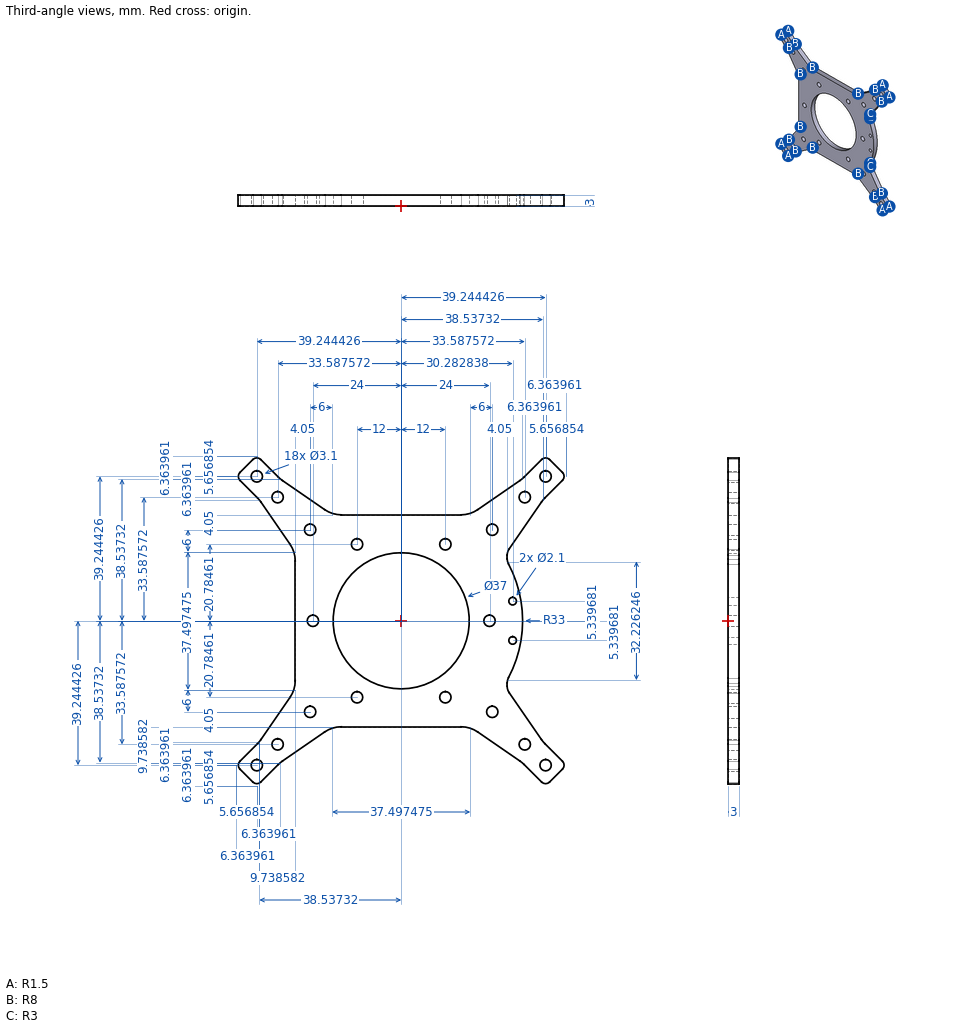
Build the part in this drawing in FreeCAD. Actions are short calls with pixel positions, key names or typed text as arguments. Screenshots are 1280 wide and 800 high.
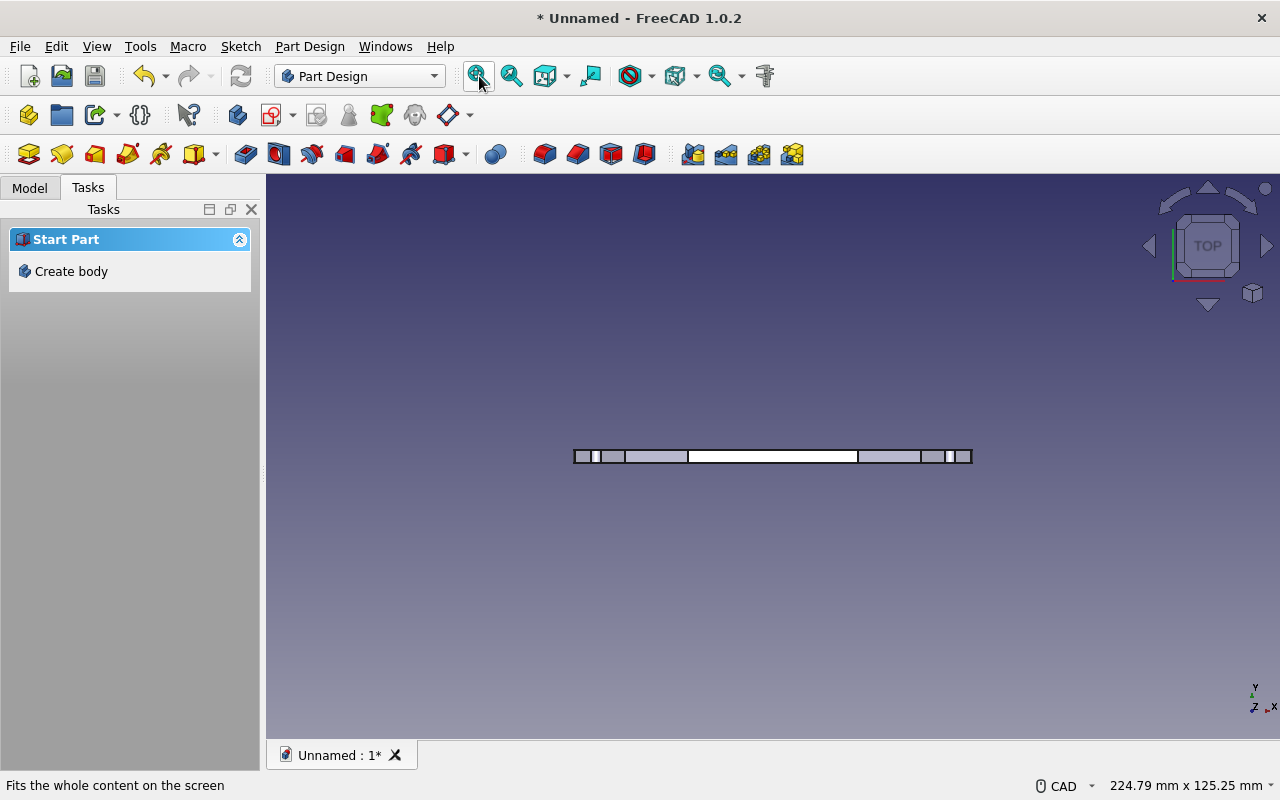
click(479, 76)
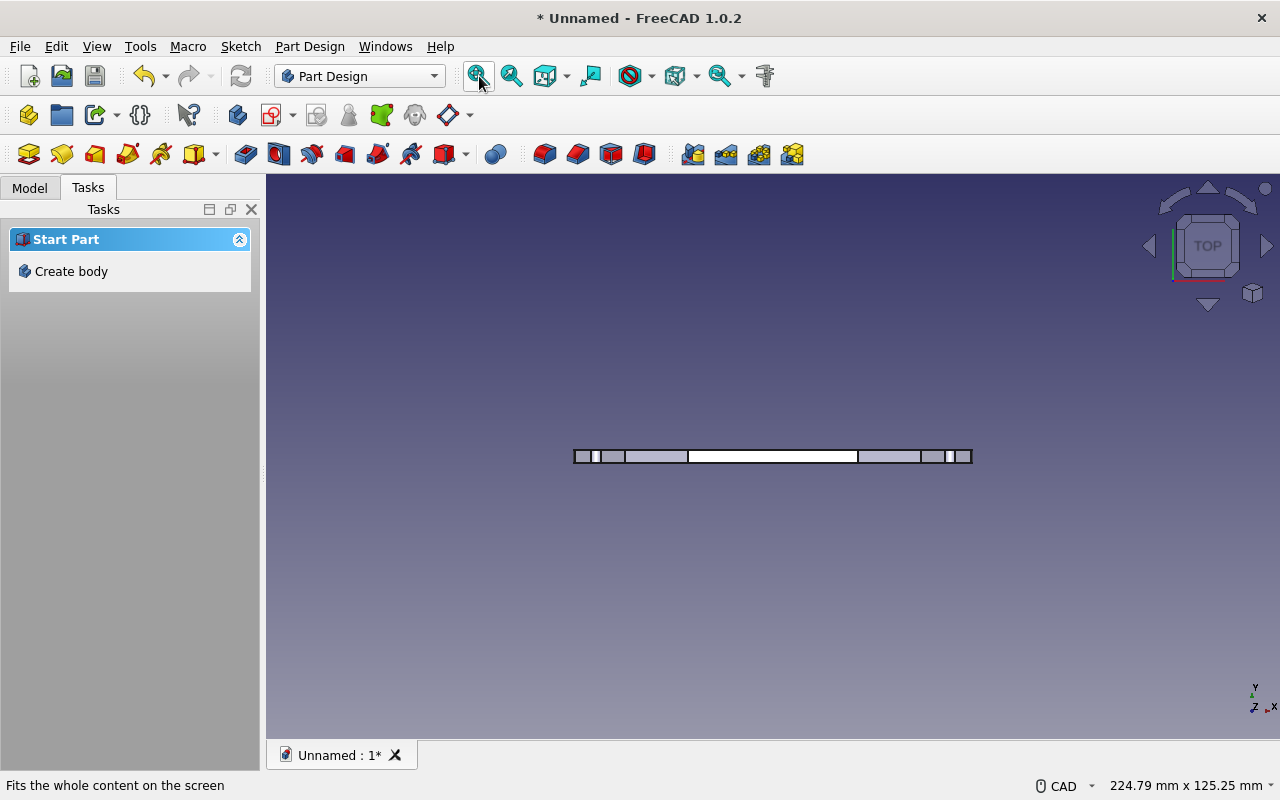
scroll(858, 455, up, 6)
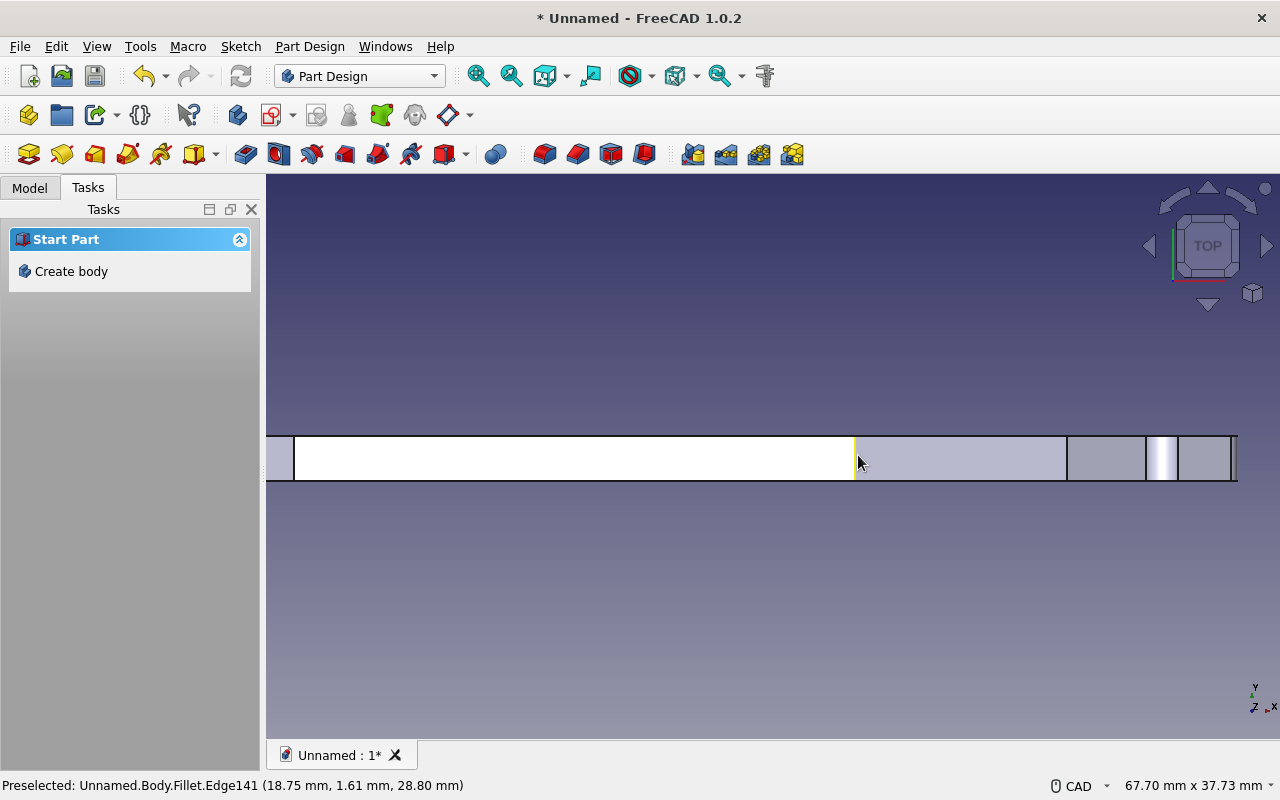
click(479, 76)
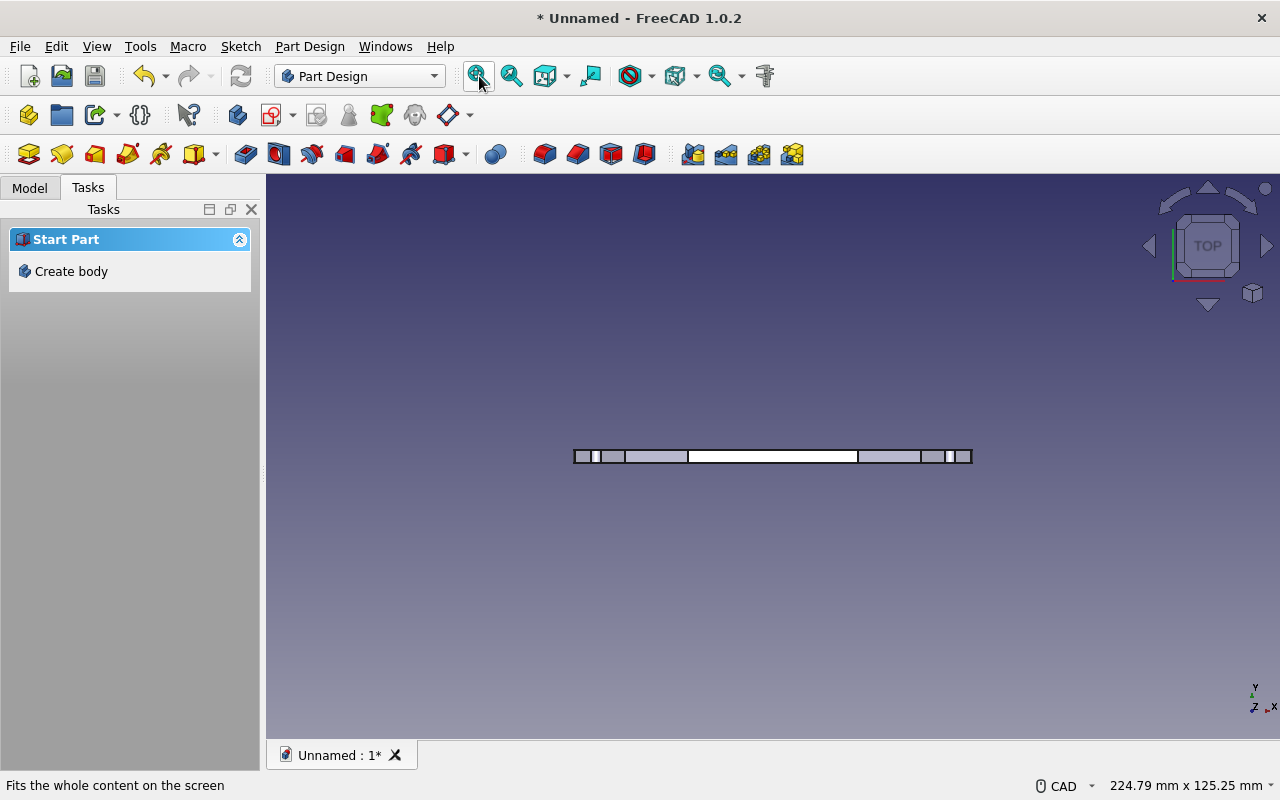
key(1)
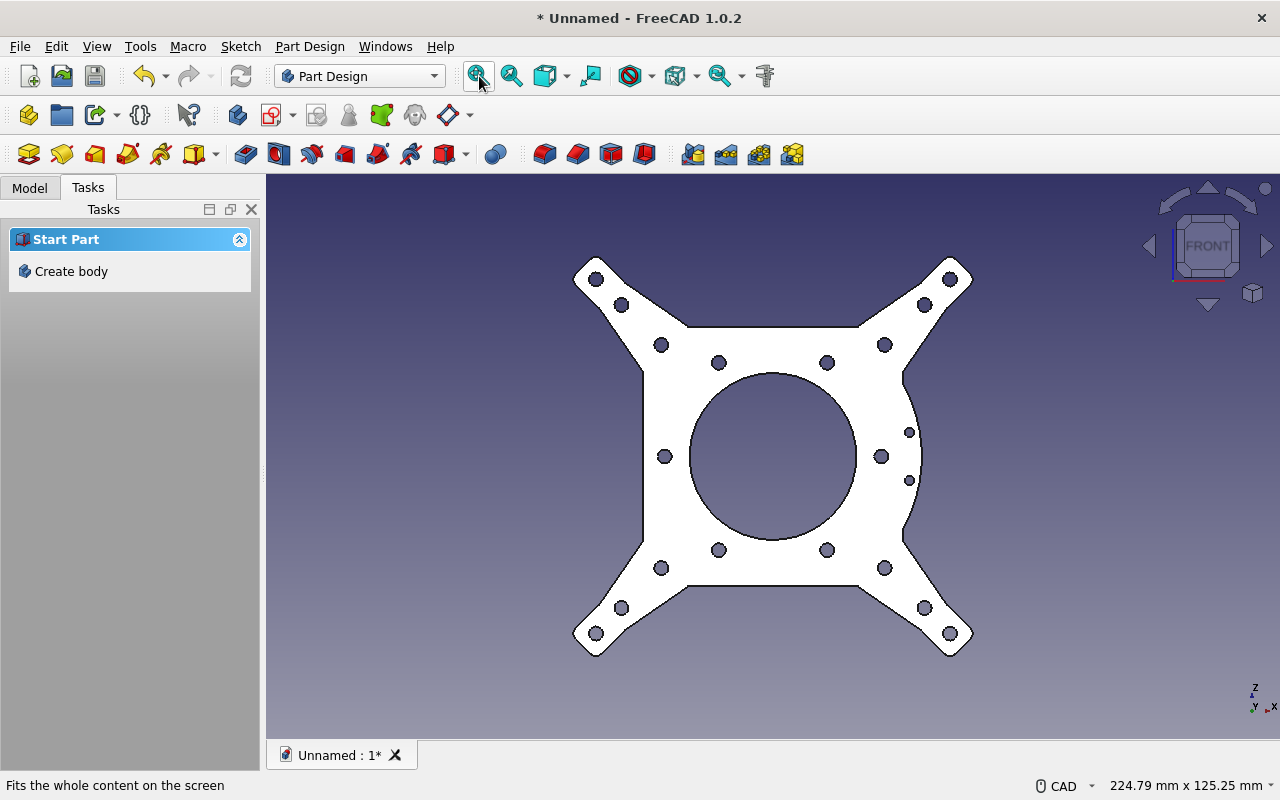
scroll(858, 585, up, 6)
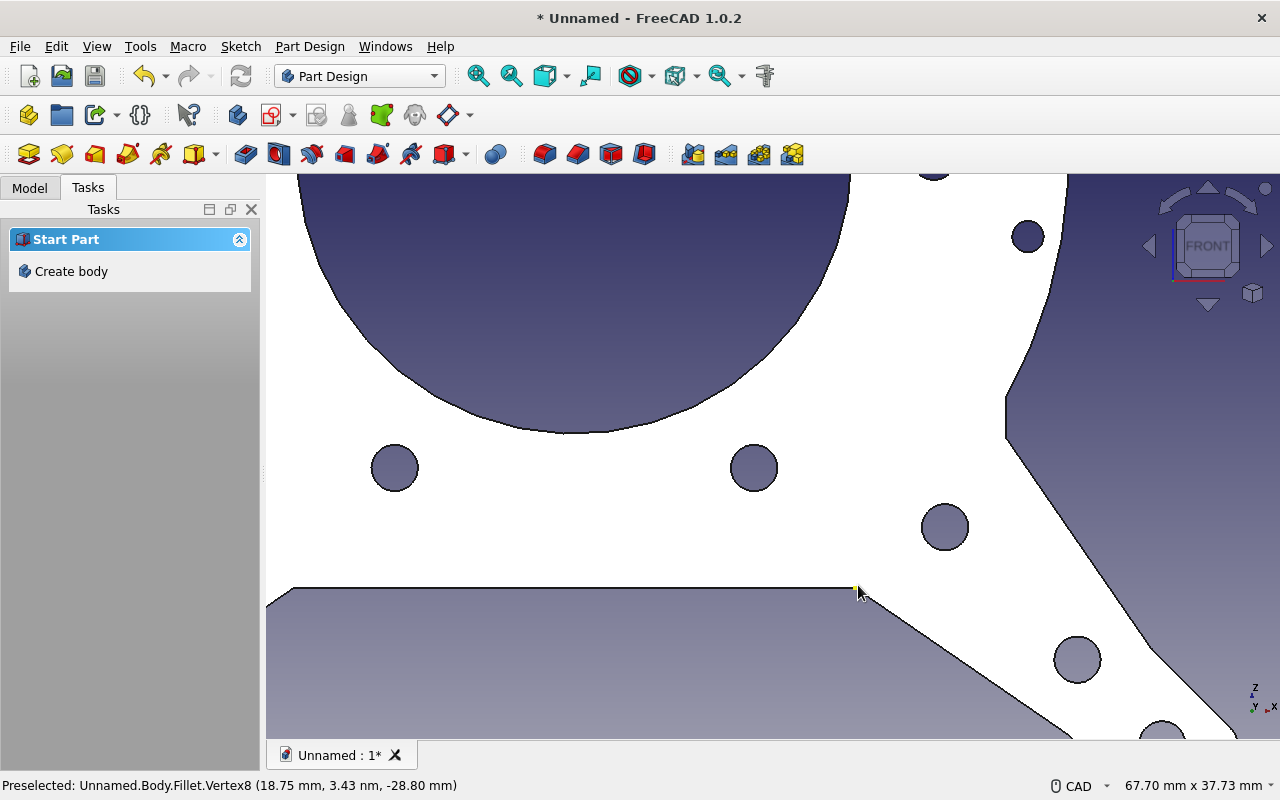
click(479, 76)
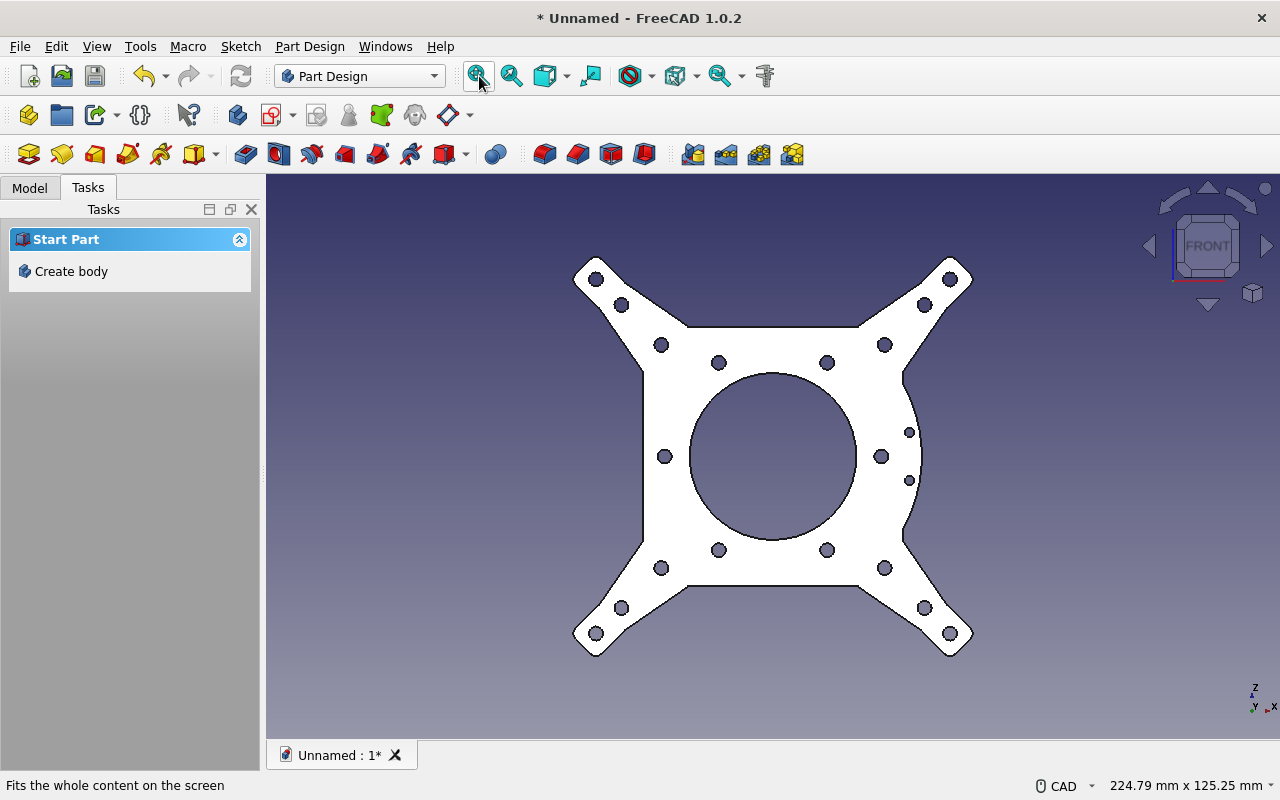
key(3)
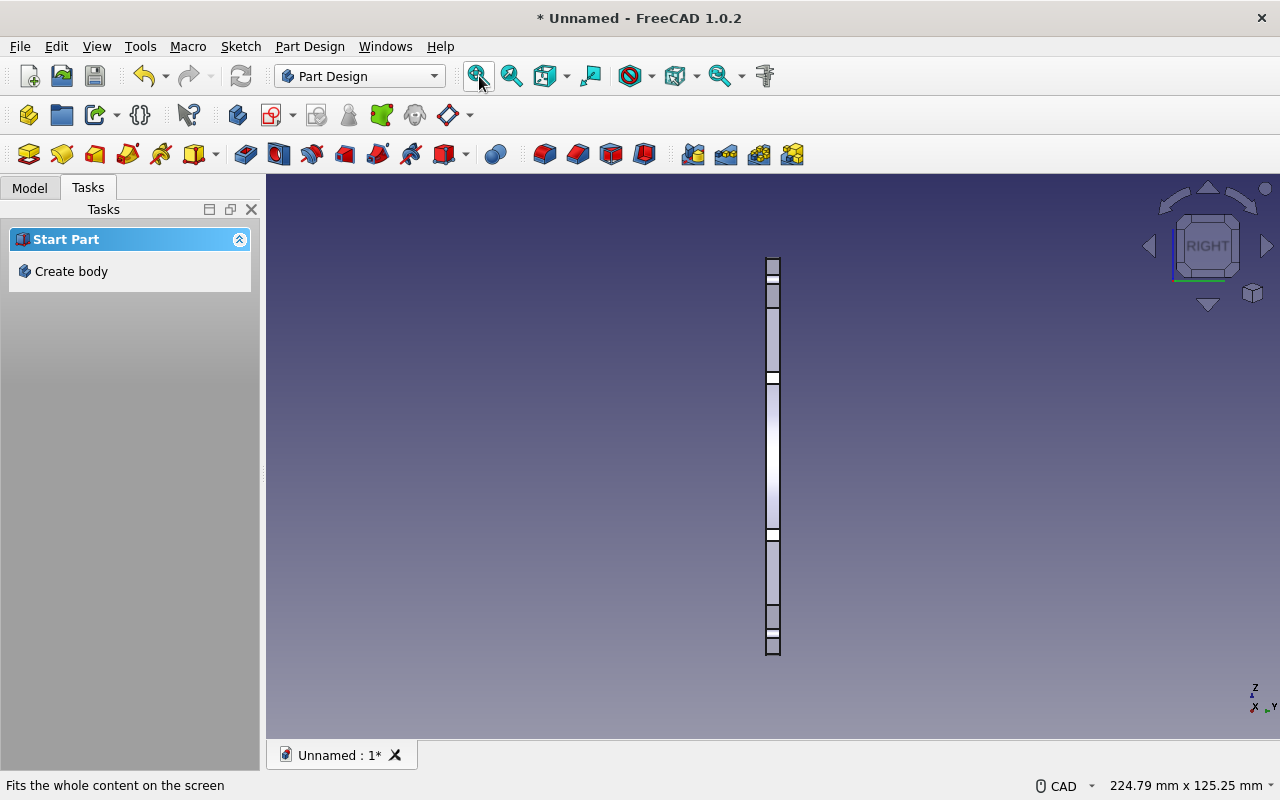
scroll(773, 585, up, 6)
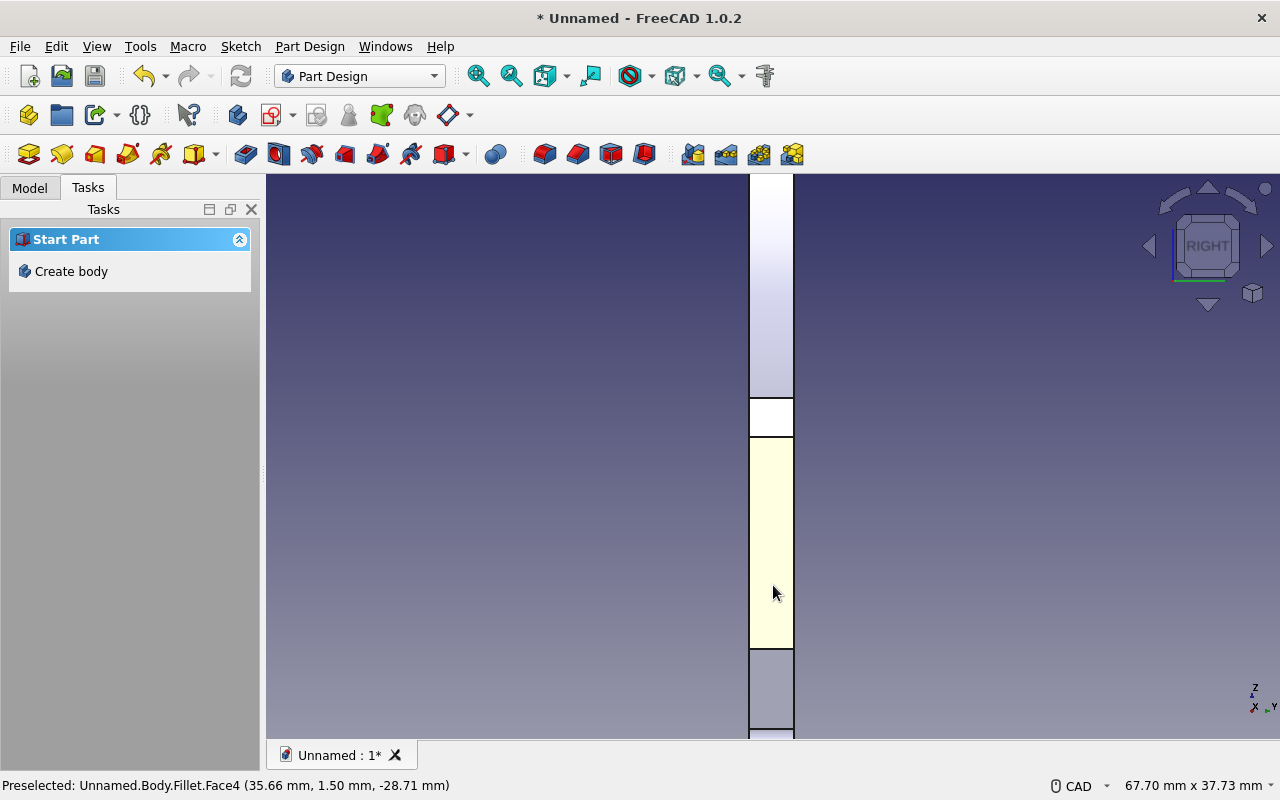
click(479, 76)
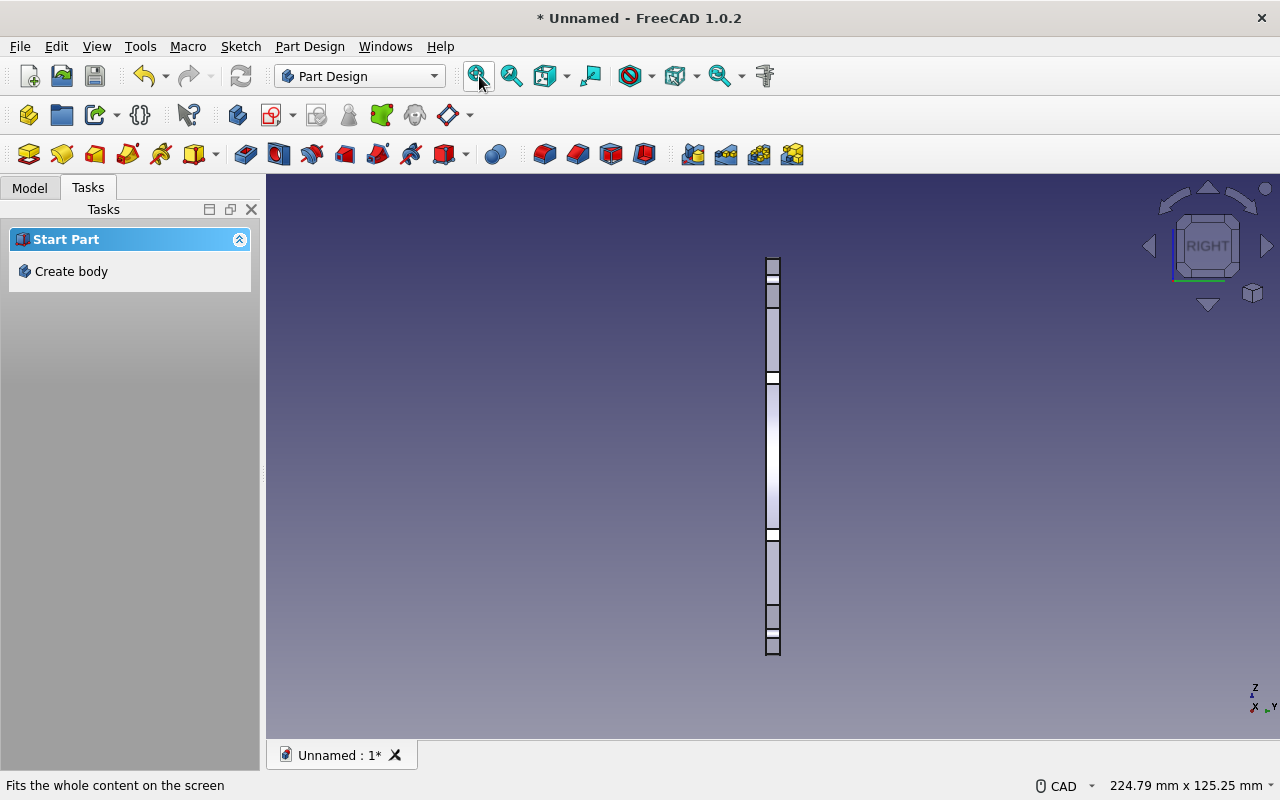
key(5)